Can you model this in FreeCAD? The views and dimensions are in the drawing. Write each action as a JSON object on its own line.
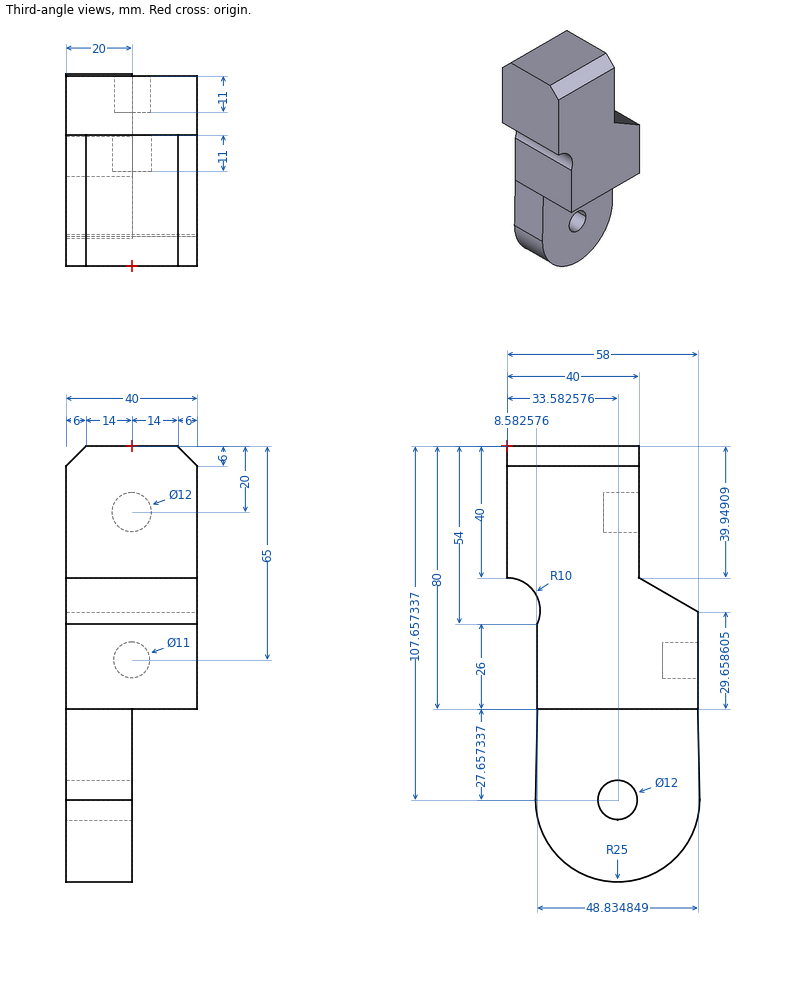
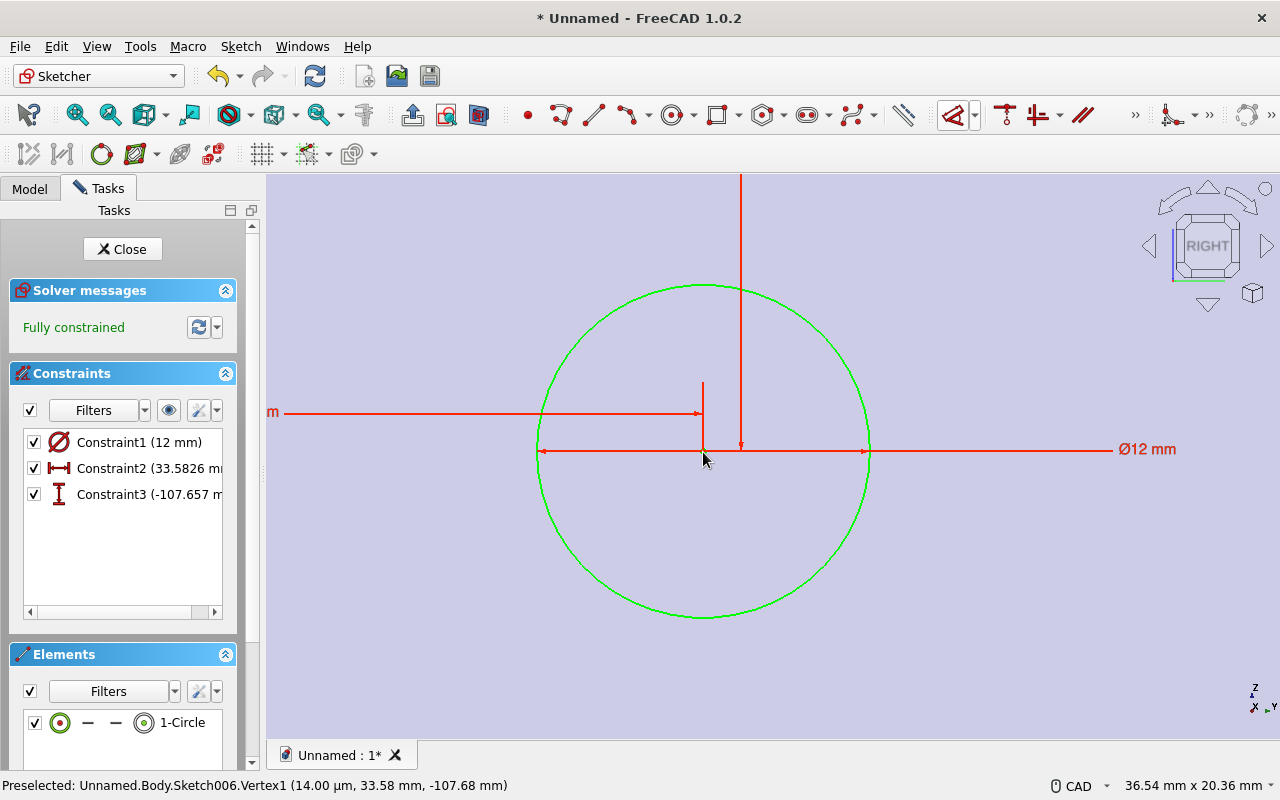
{"action": "left_click", "coordinate": [123, 249]}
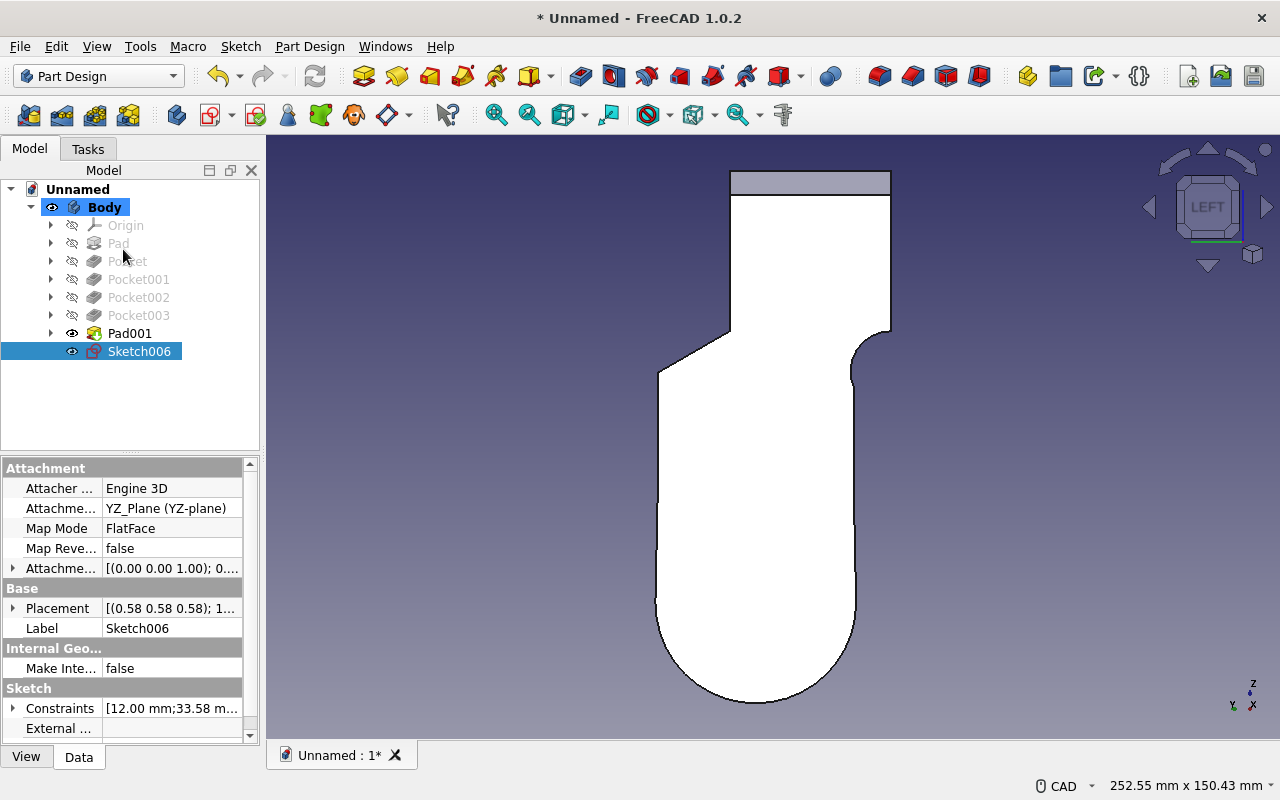
{"action": "left_click", "coordinate": [581, 76]}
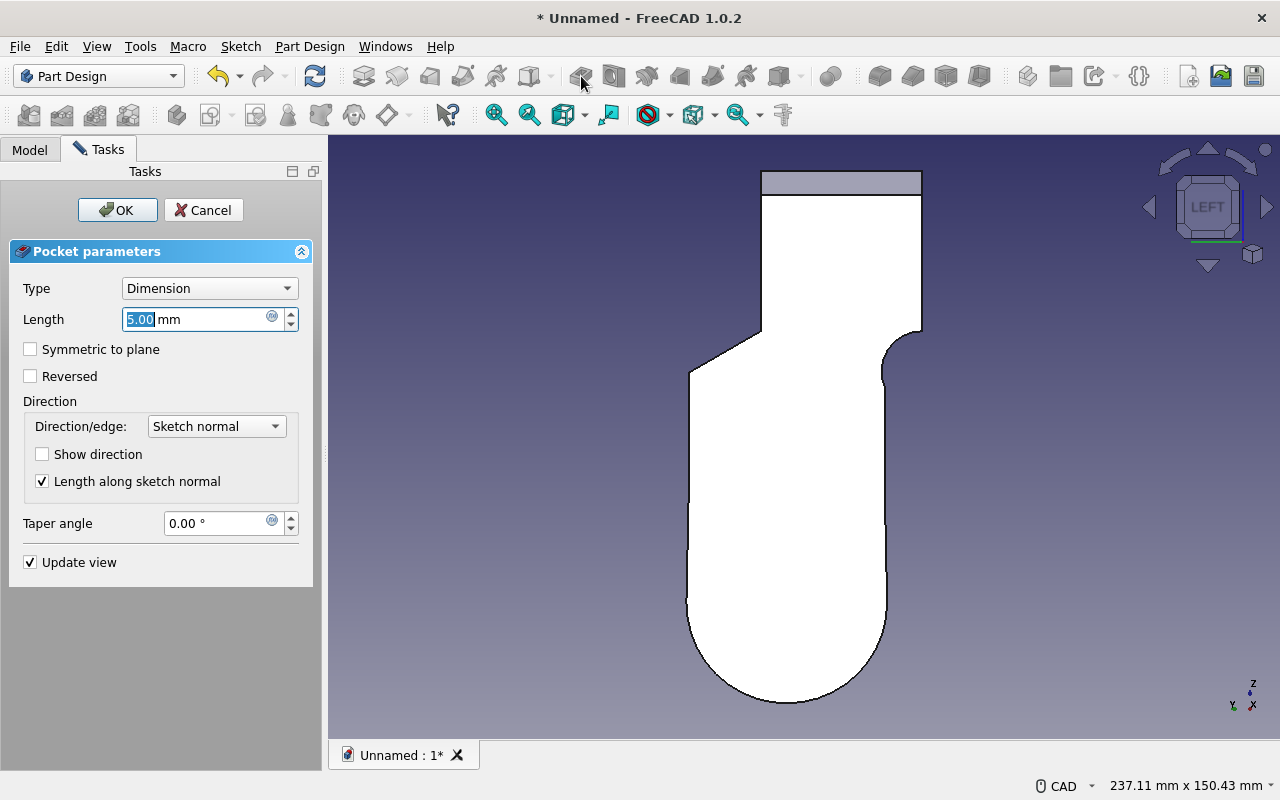
{"action": "left_click", "coordinate": [210, 288]}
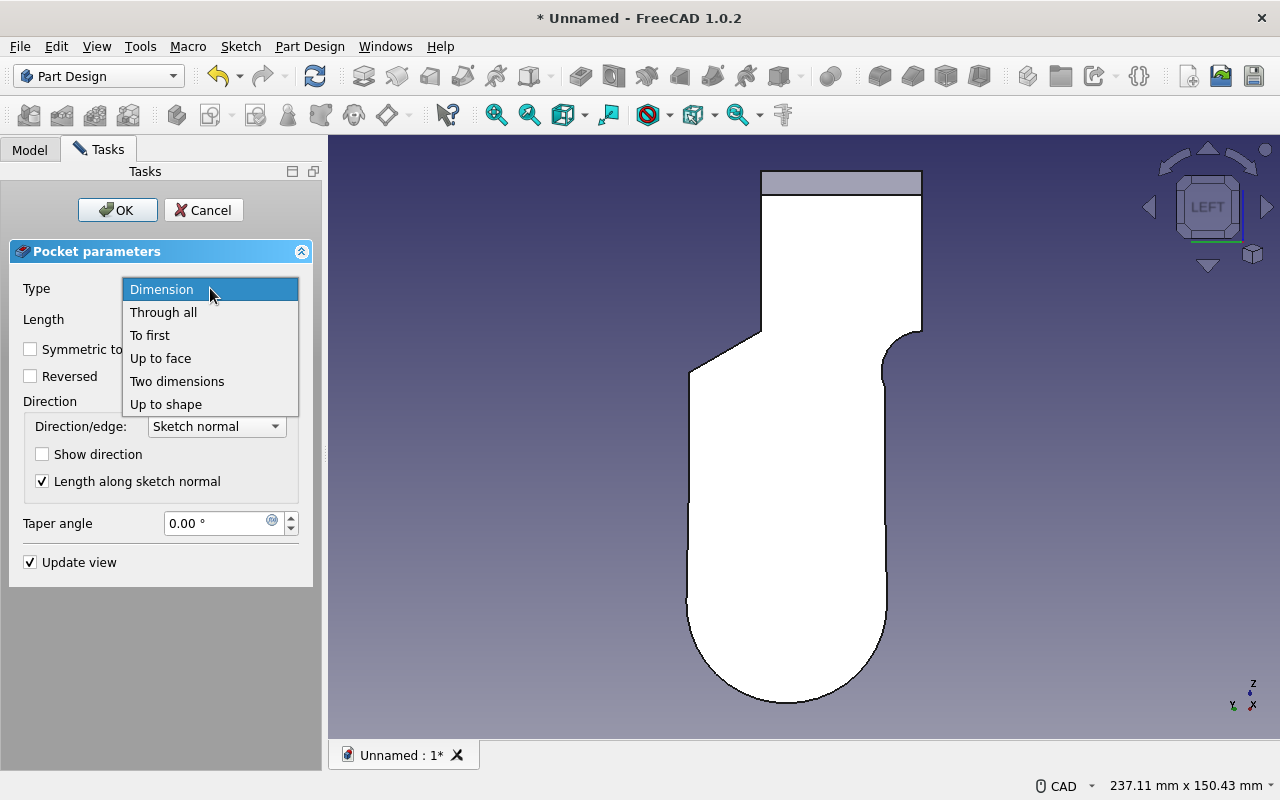
{"action": "left_click", "coordinate": [208, 312]}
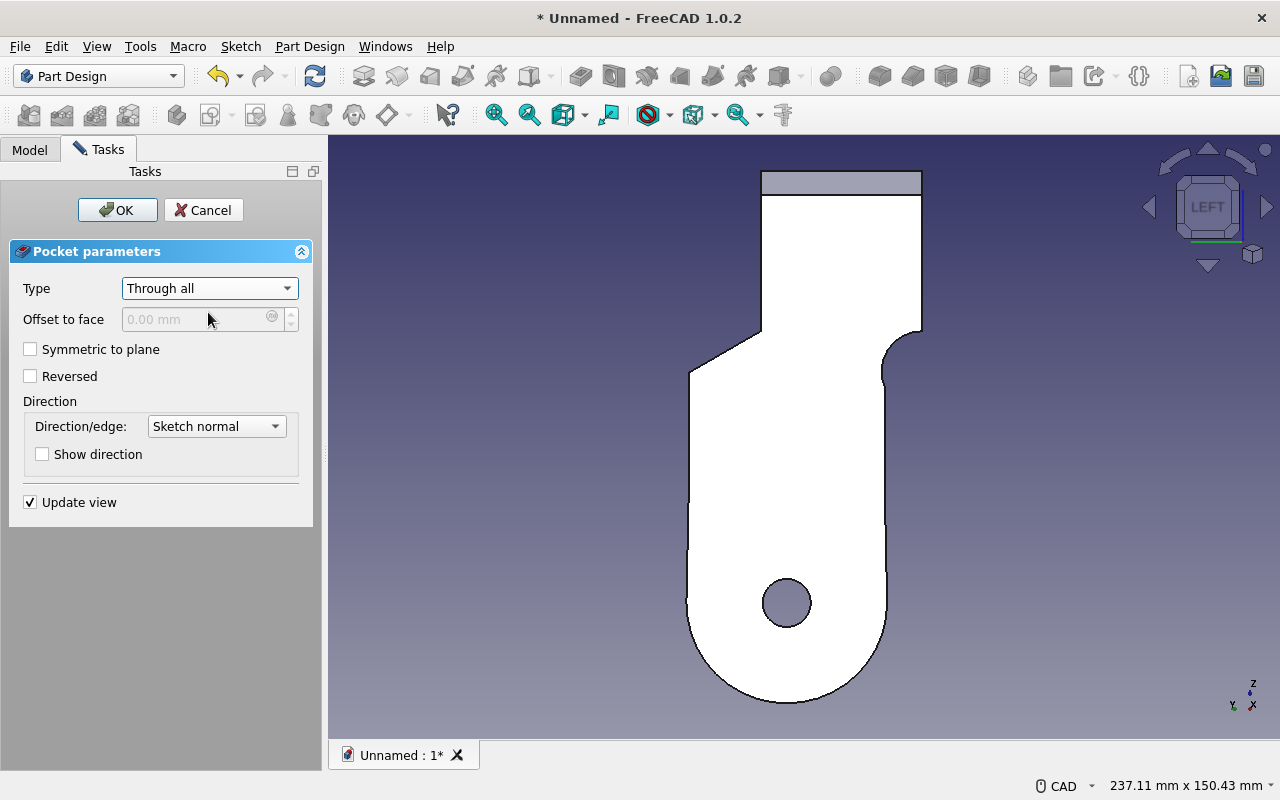
{"action": "left_click", "coordinate": [118, 210]}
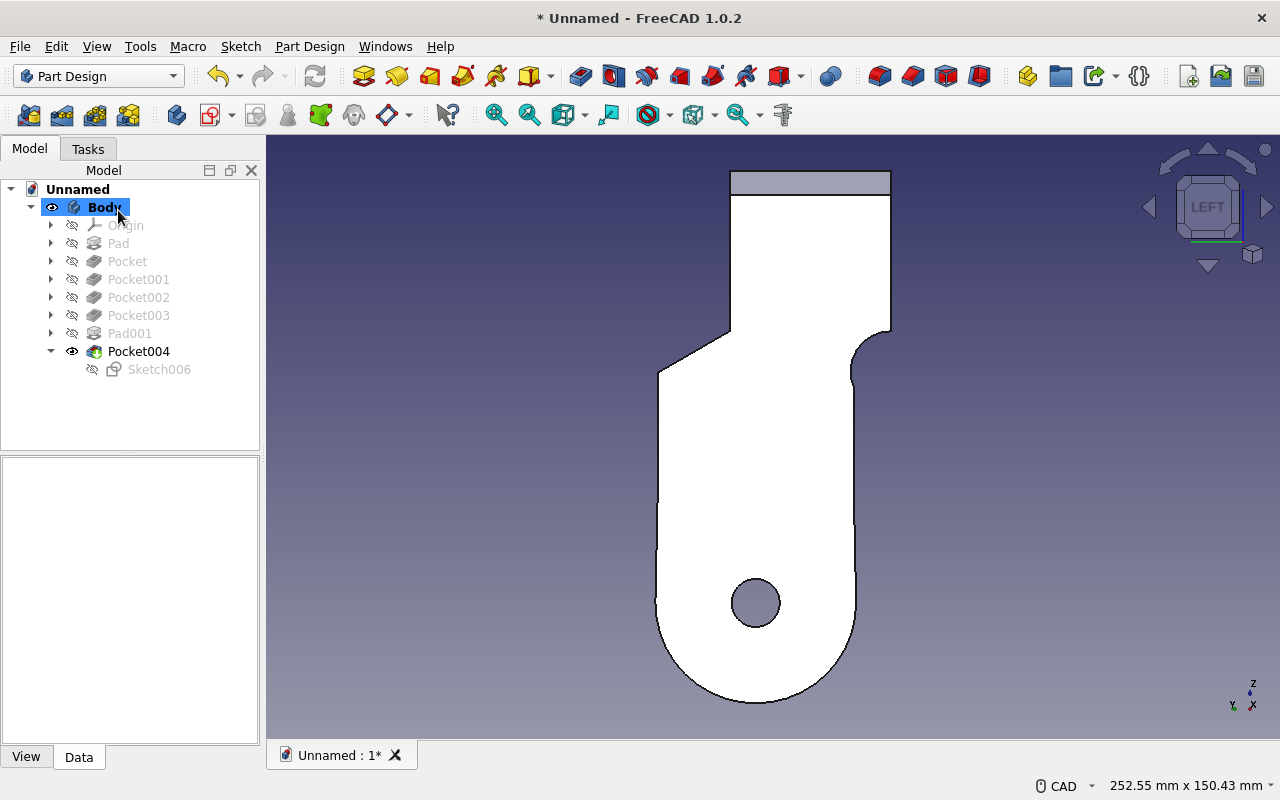
{"action": "key", "text": "0"}